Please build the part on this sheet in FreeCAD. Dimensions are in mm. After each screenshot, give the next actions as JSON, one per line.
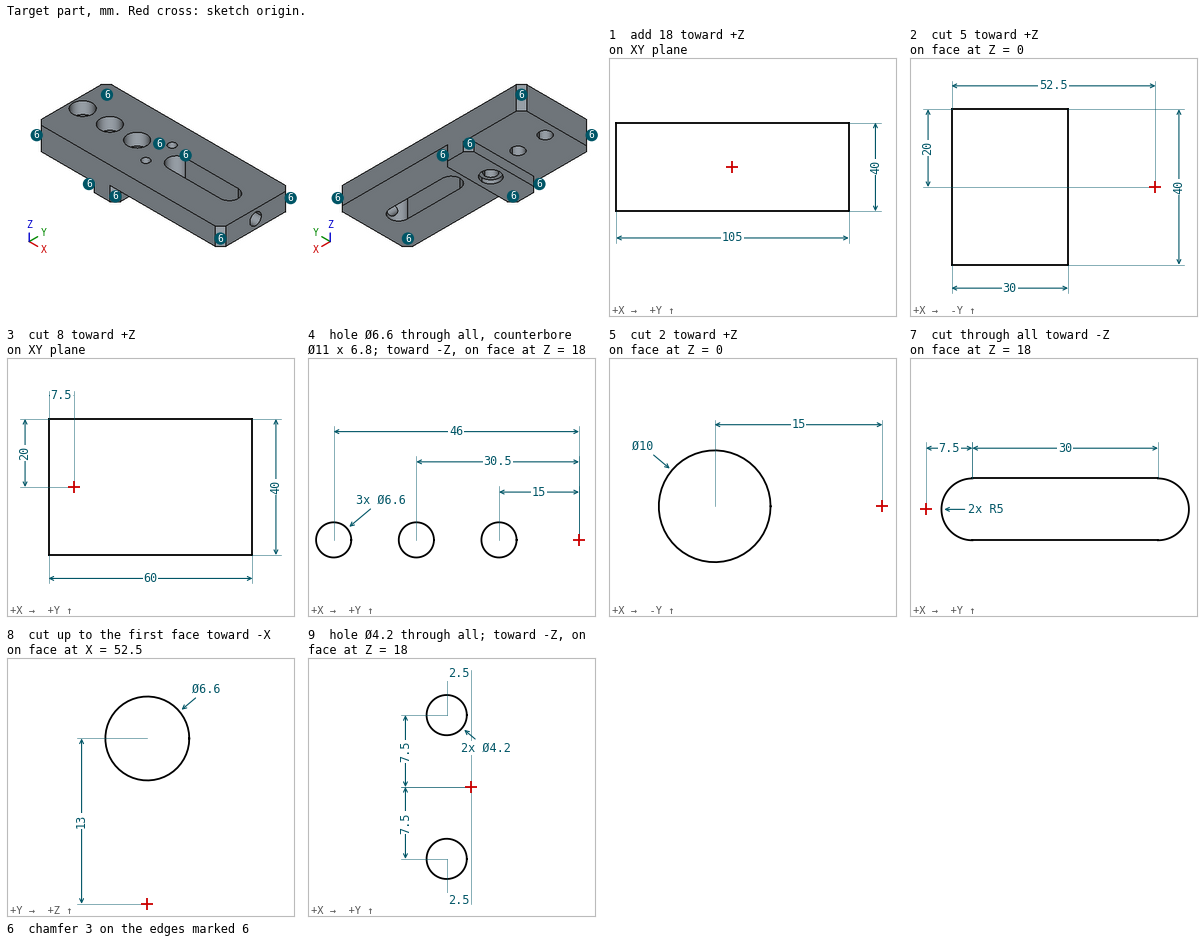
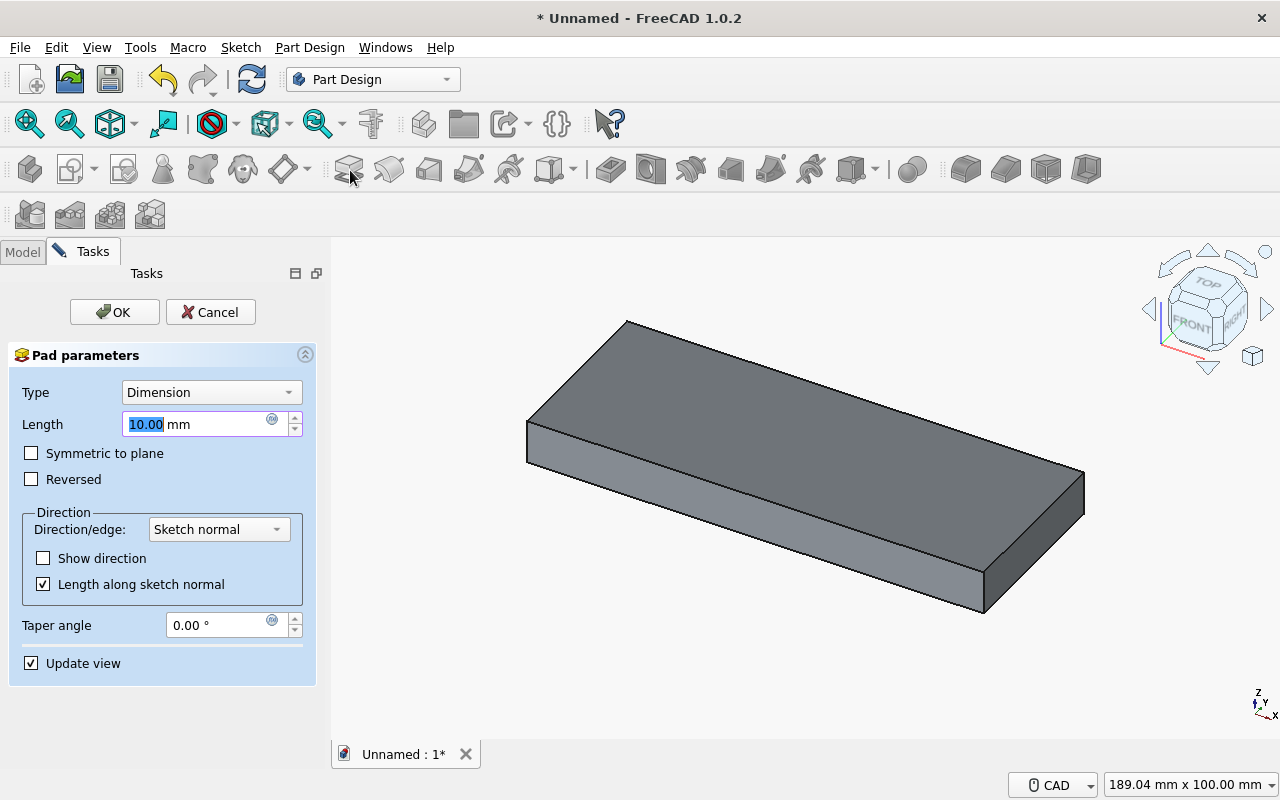
{"action": "type", "text": "18"}
{"action": "key", "text": "Tab"}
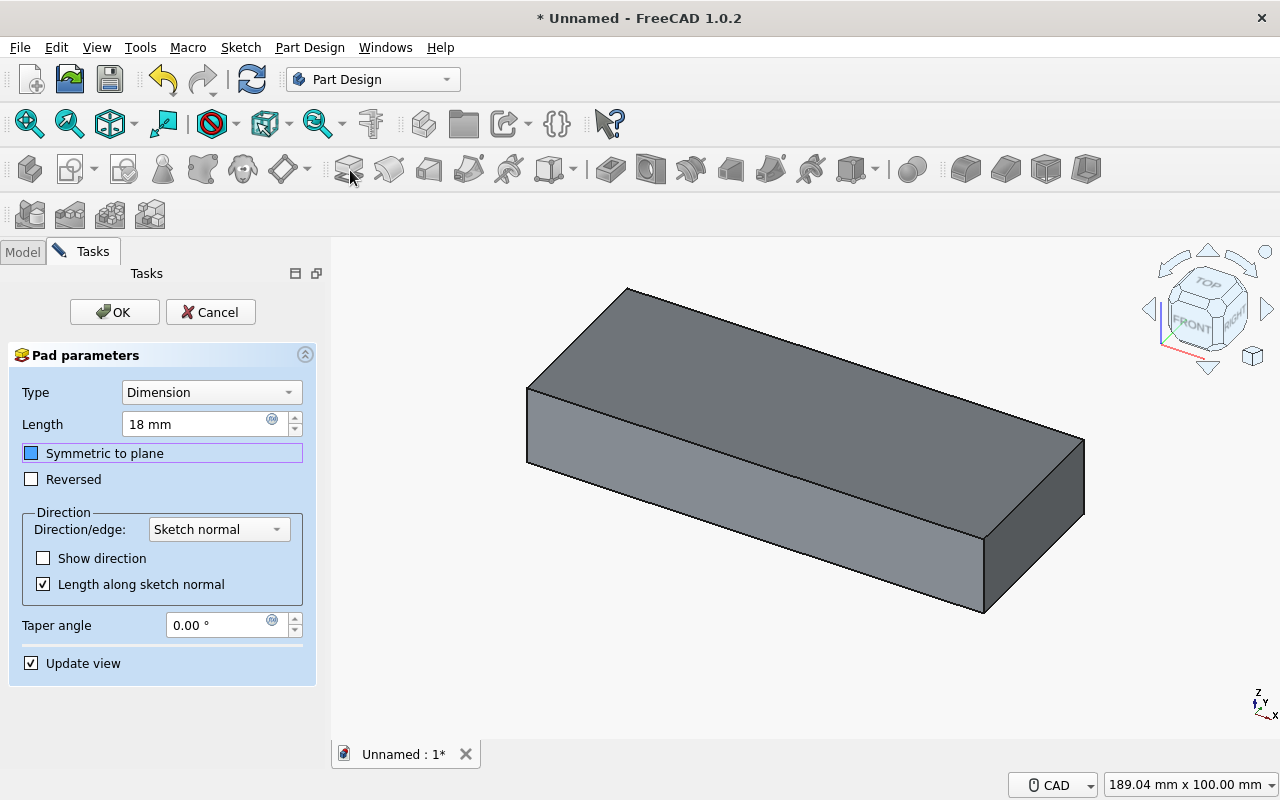
{"action": "left_click", "coordinate": [115, 312]}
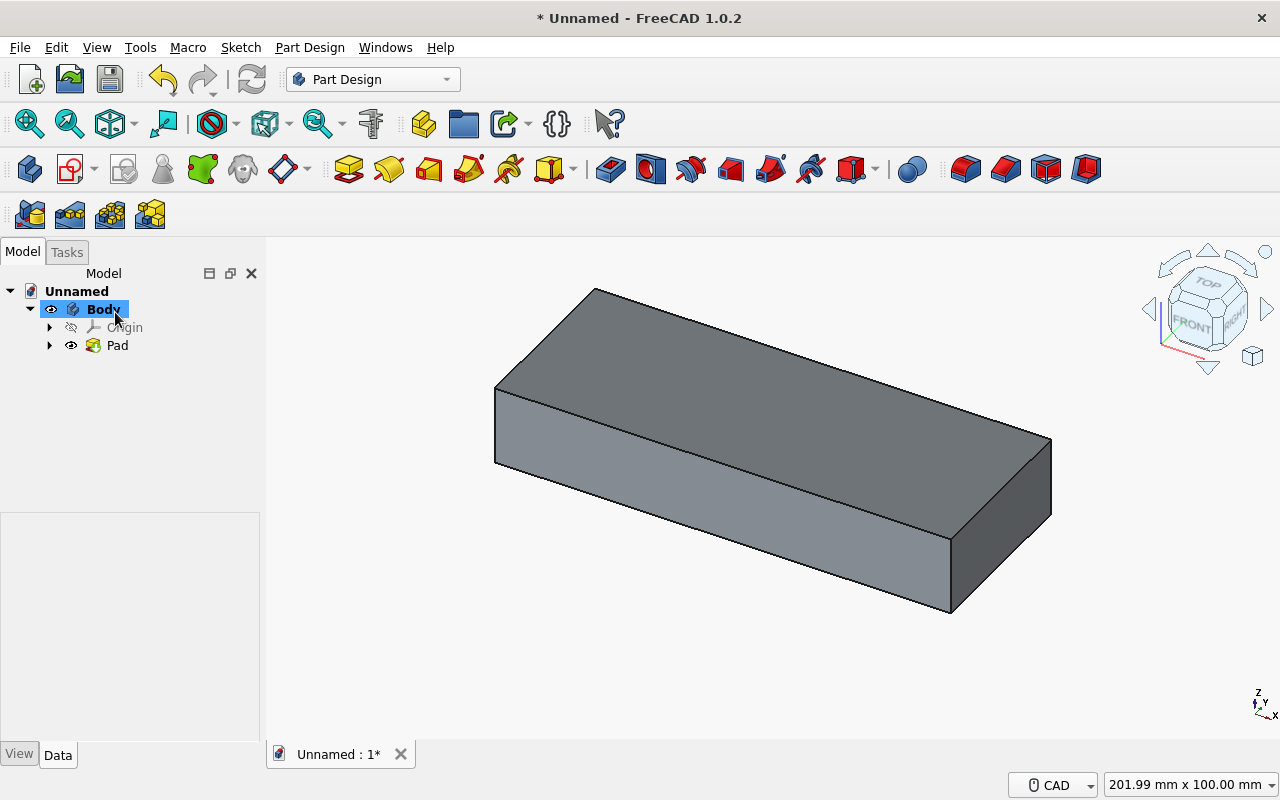
{"action": "key", "text": "5"}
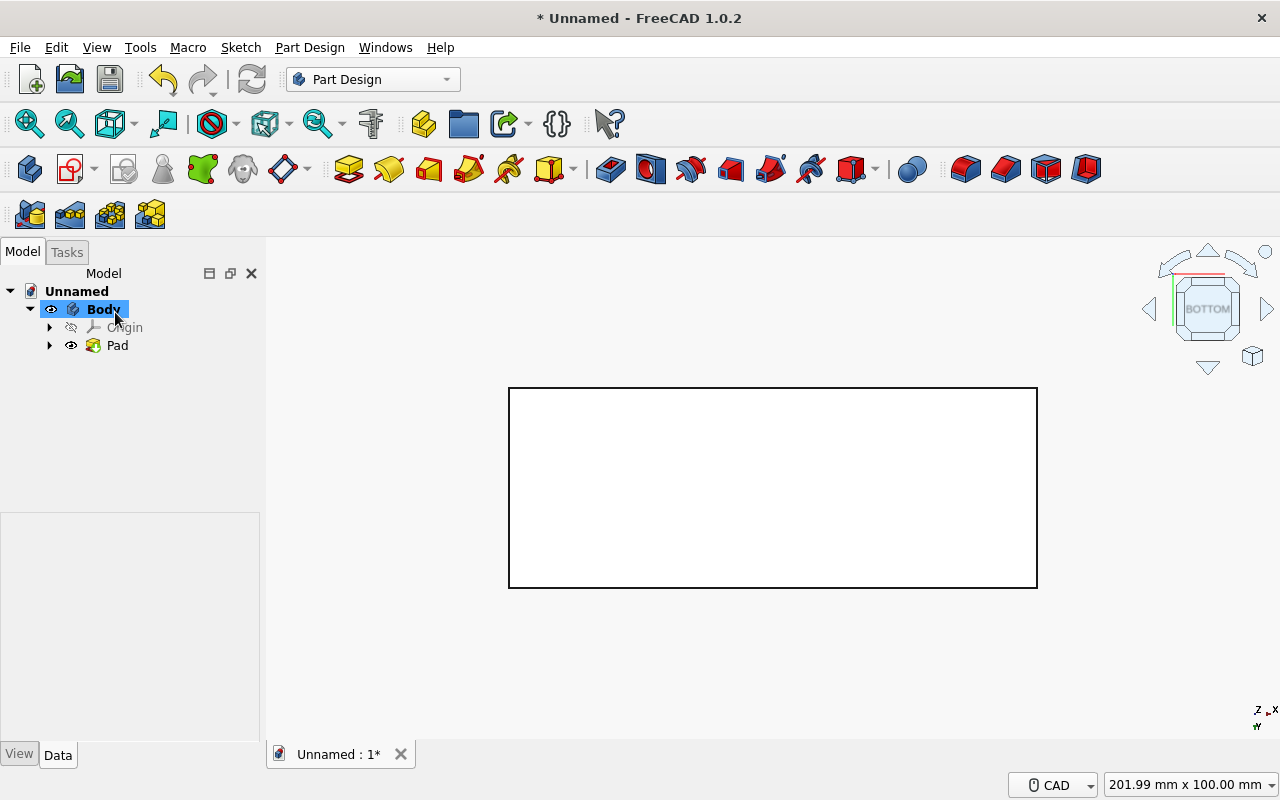
{"action": "left_click", "coordinate": [924, 487]}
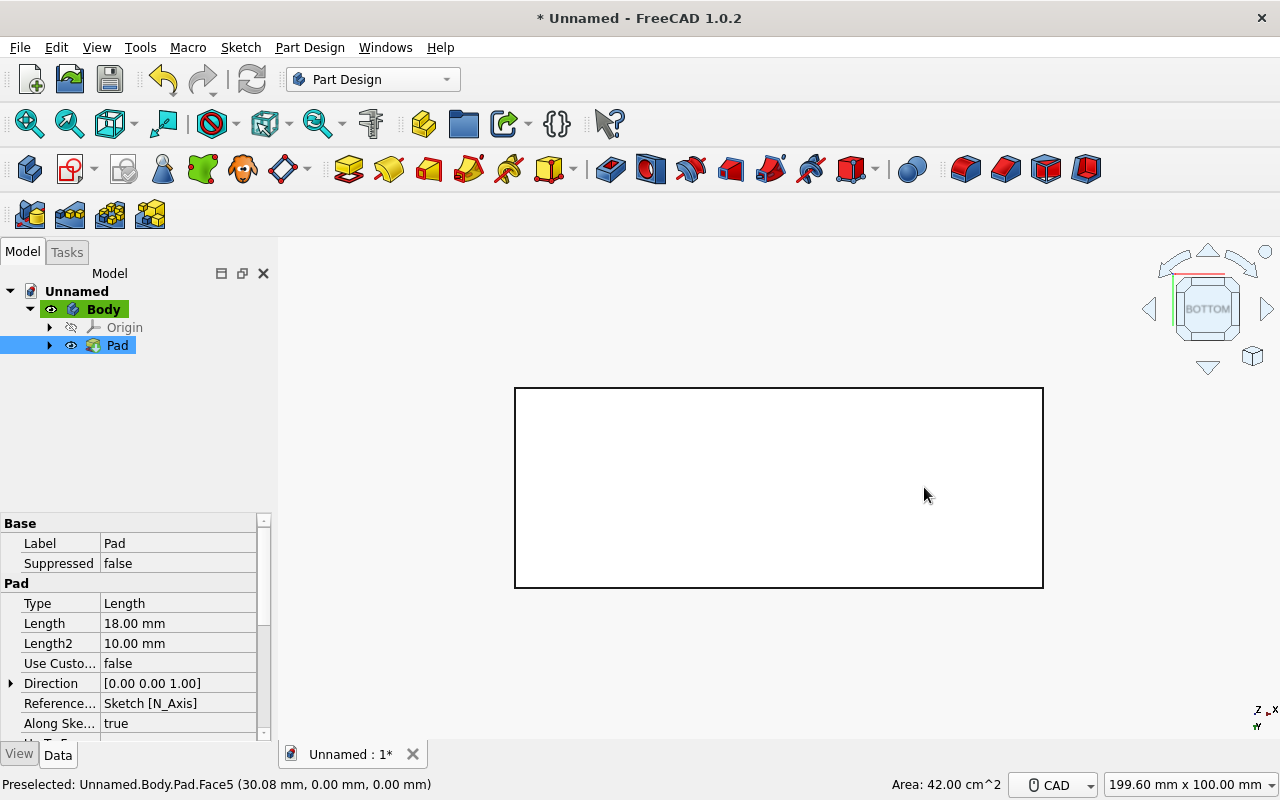
{"action": "left_click", "coordinate": [70, 170]}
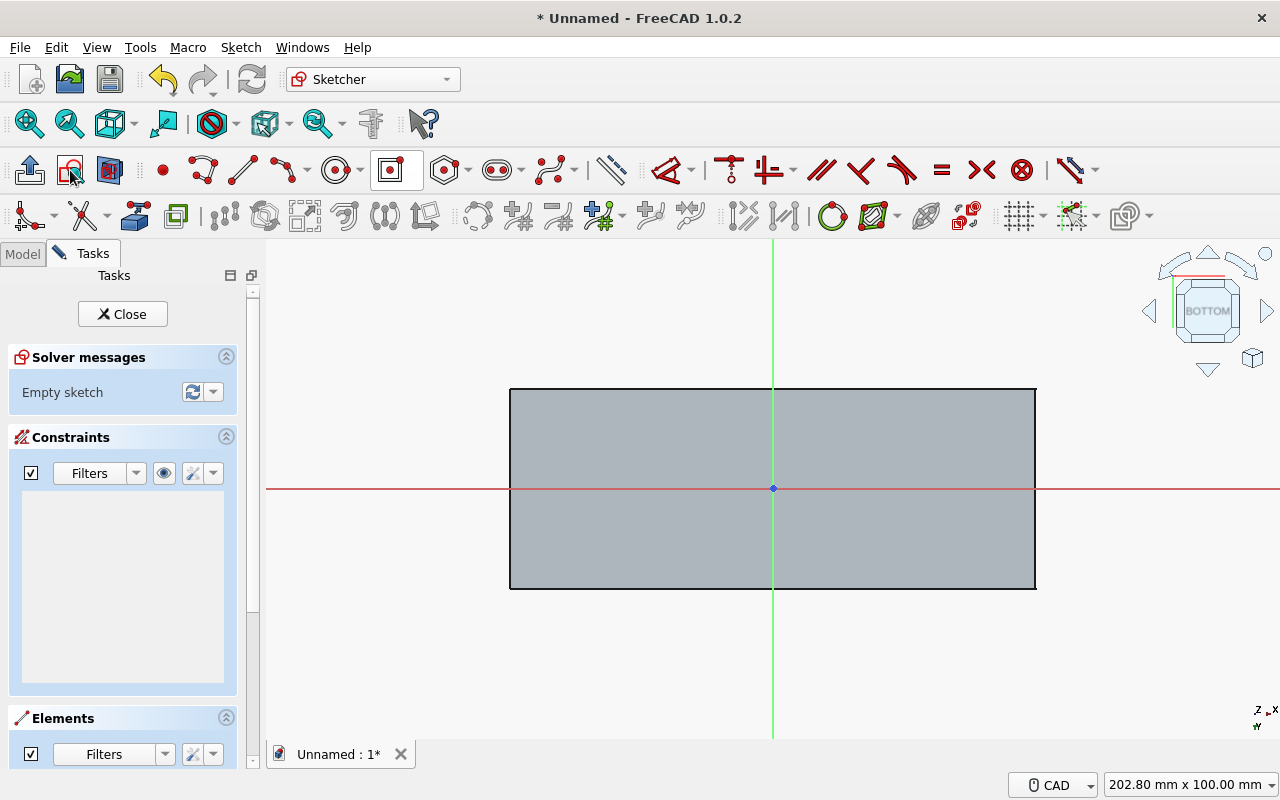
{"action": "scroll", "coordinate": [514, 489], "scroll_direction": "up", "scroll_amount": 2}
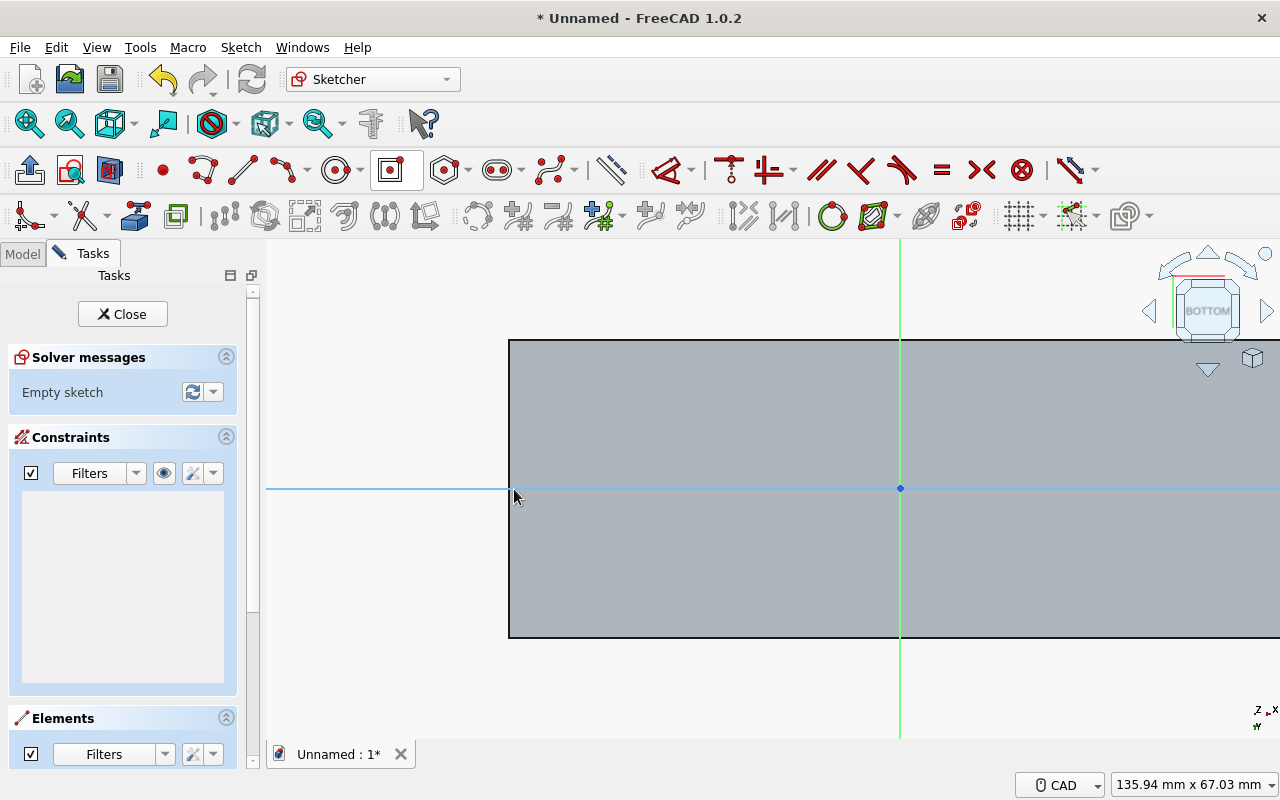
{"action": "key", "text": "g r"}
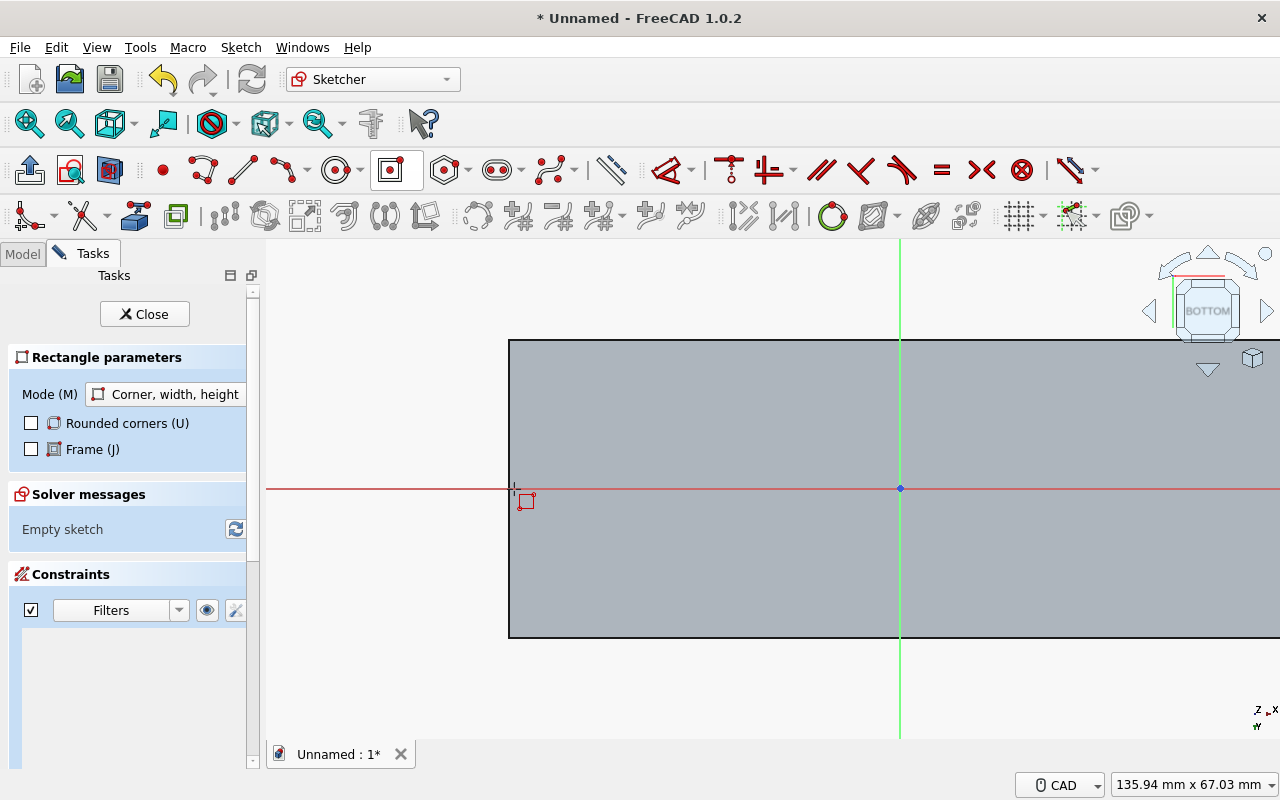
{"action": "left_click", "coordinate": [509, 340]}
{"action": "mouse_move", "coordinate": [732, 638]}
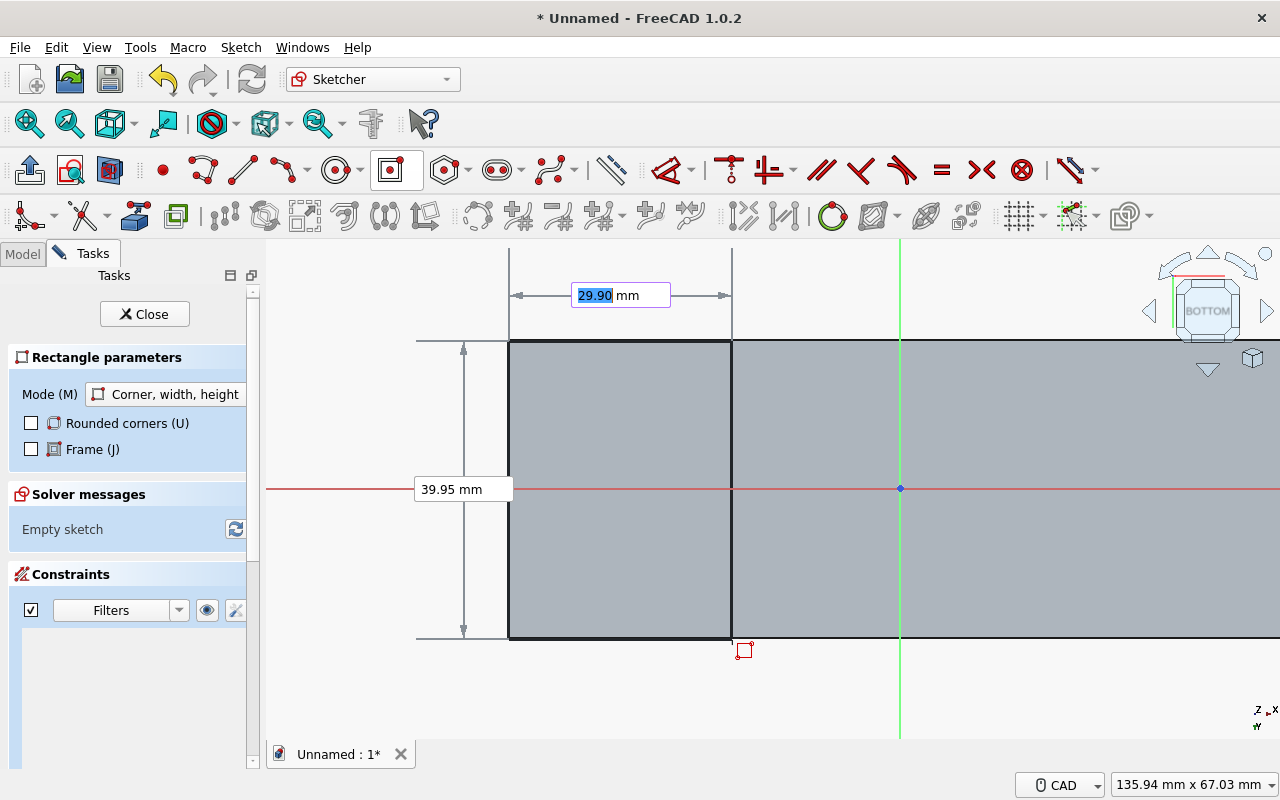
{"action": "type", "text": "30"}
{"action": "key", "text": "Tab"}
{"action": "type", "text": "40"}
{"action": "key", "text": "Return"}
{"action": "key", "text": "Escape"}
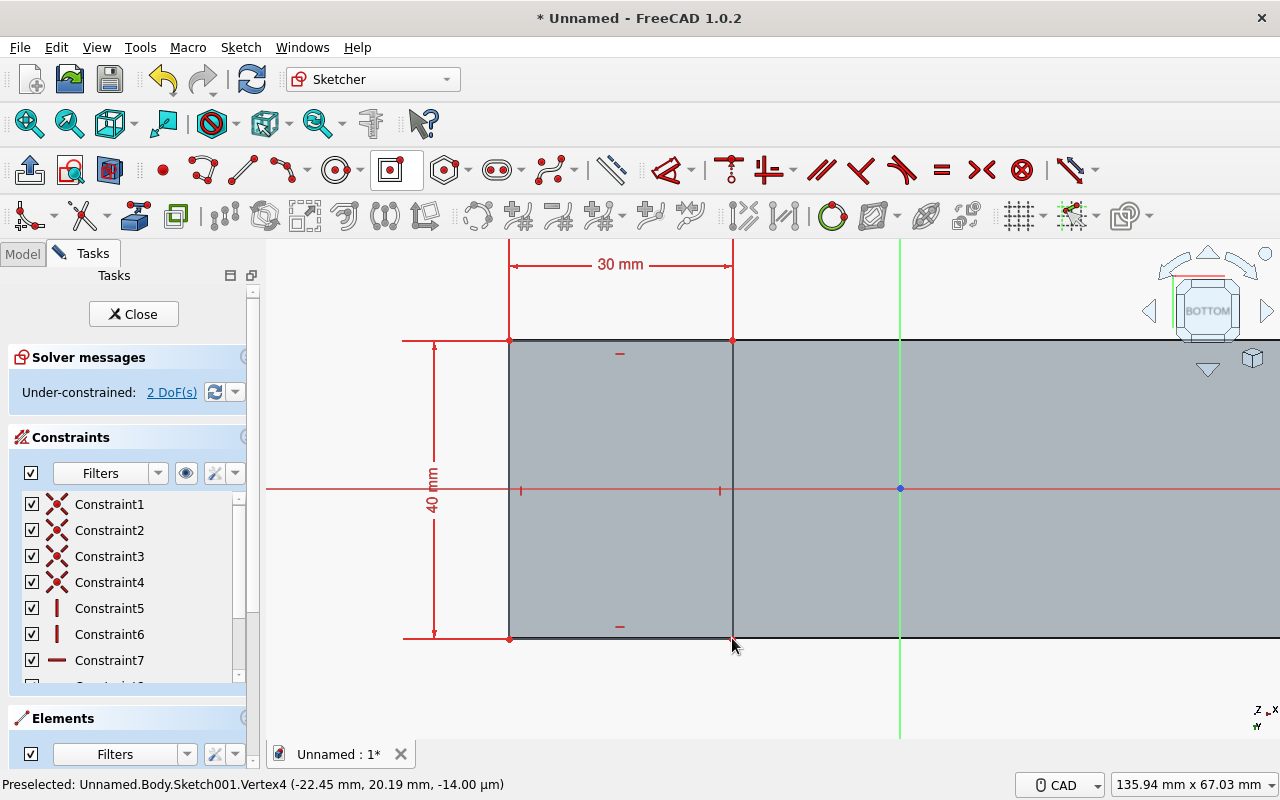
{"action": "key", "text": "d"}